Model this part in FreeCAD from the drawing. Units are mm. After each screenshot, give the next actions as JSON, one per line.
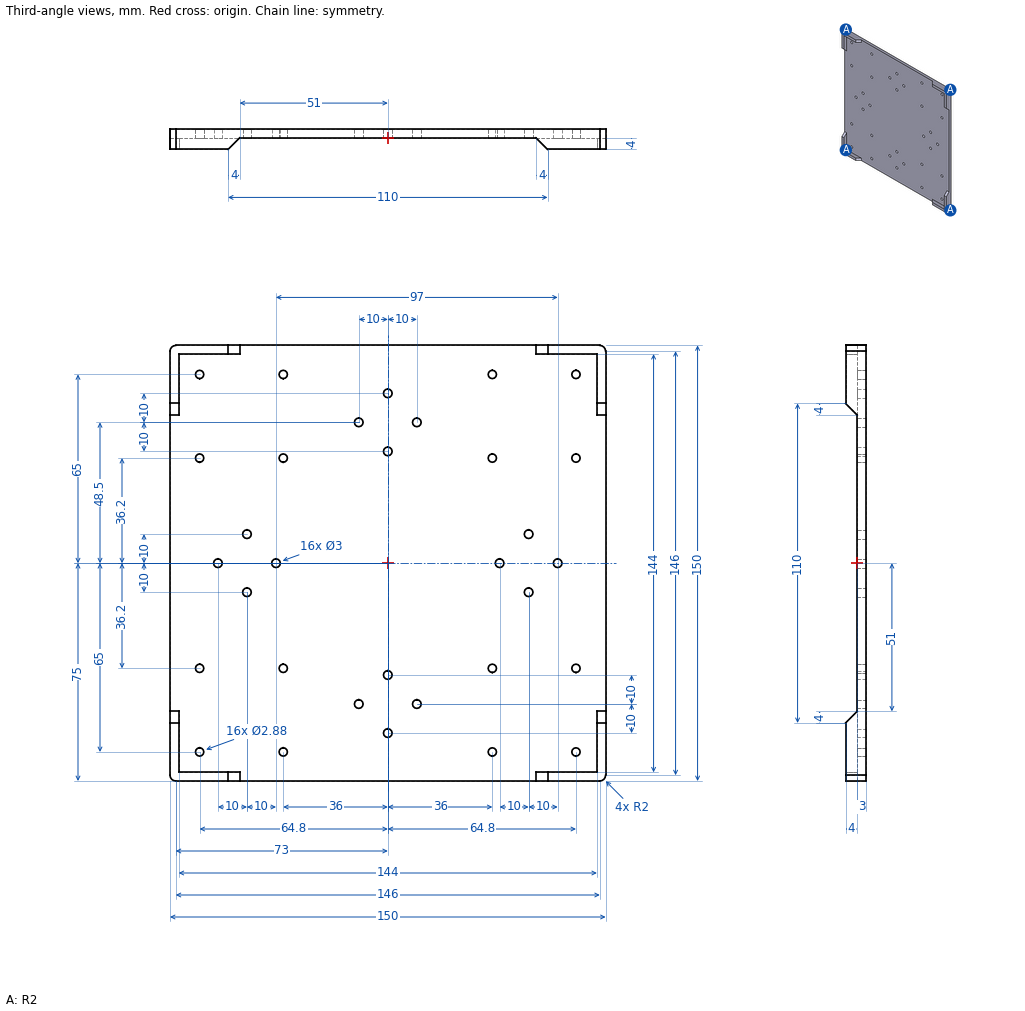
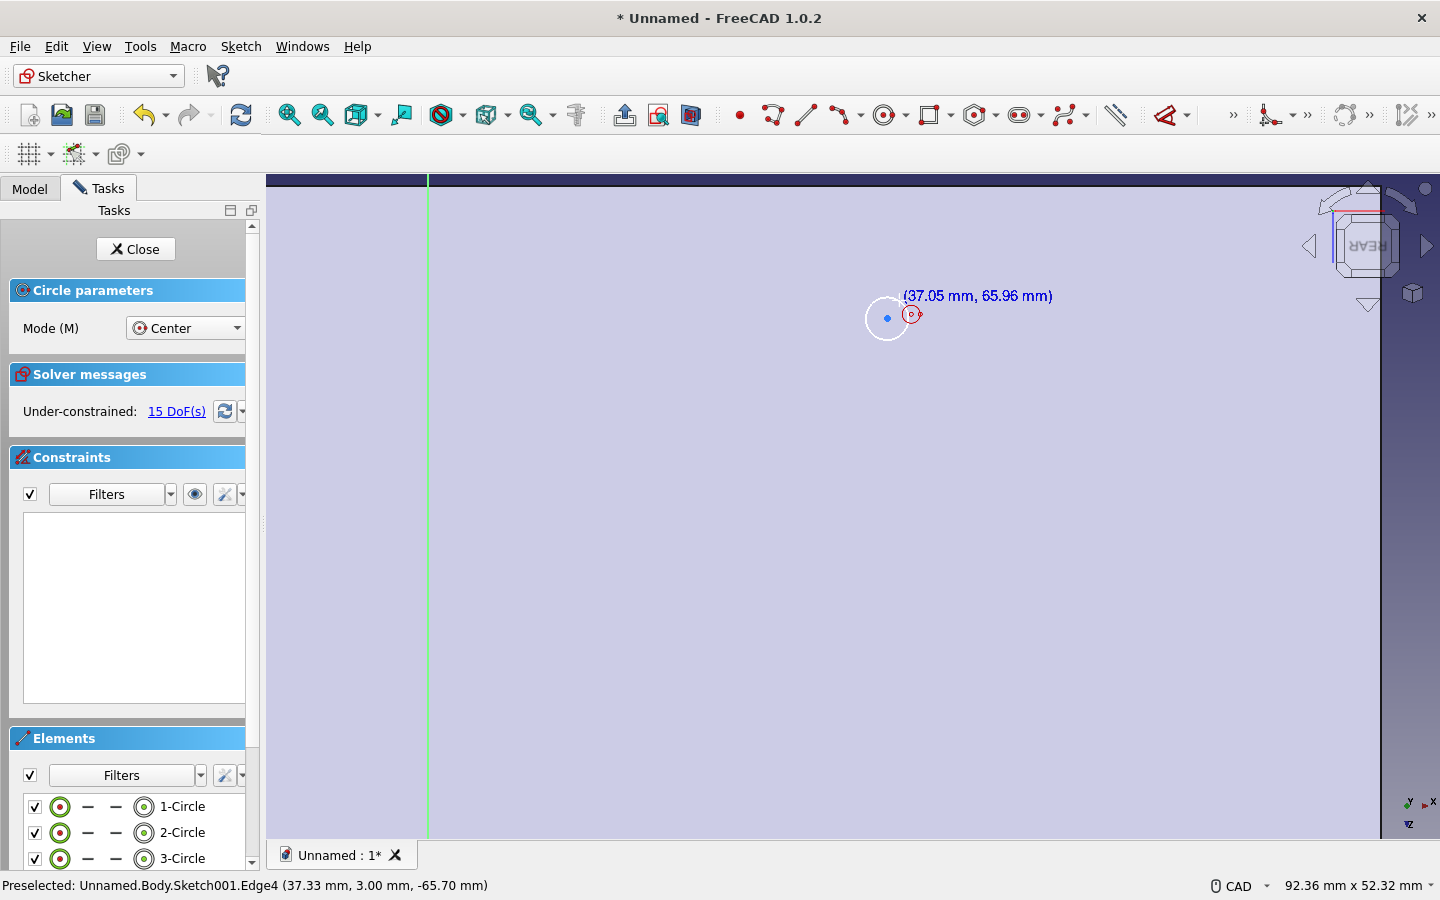
{"action": "scroll", "coordinate": [1252, 313], "scroll_direction": "up", "scroll_amount": 2}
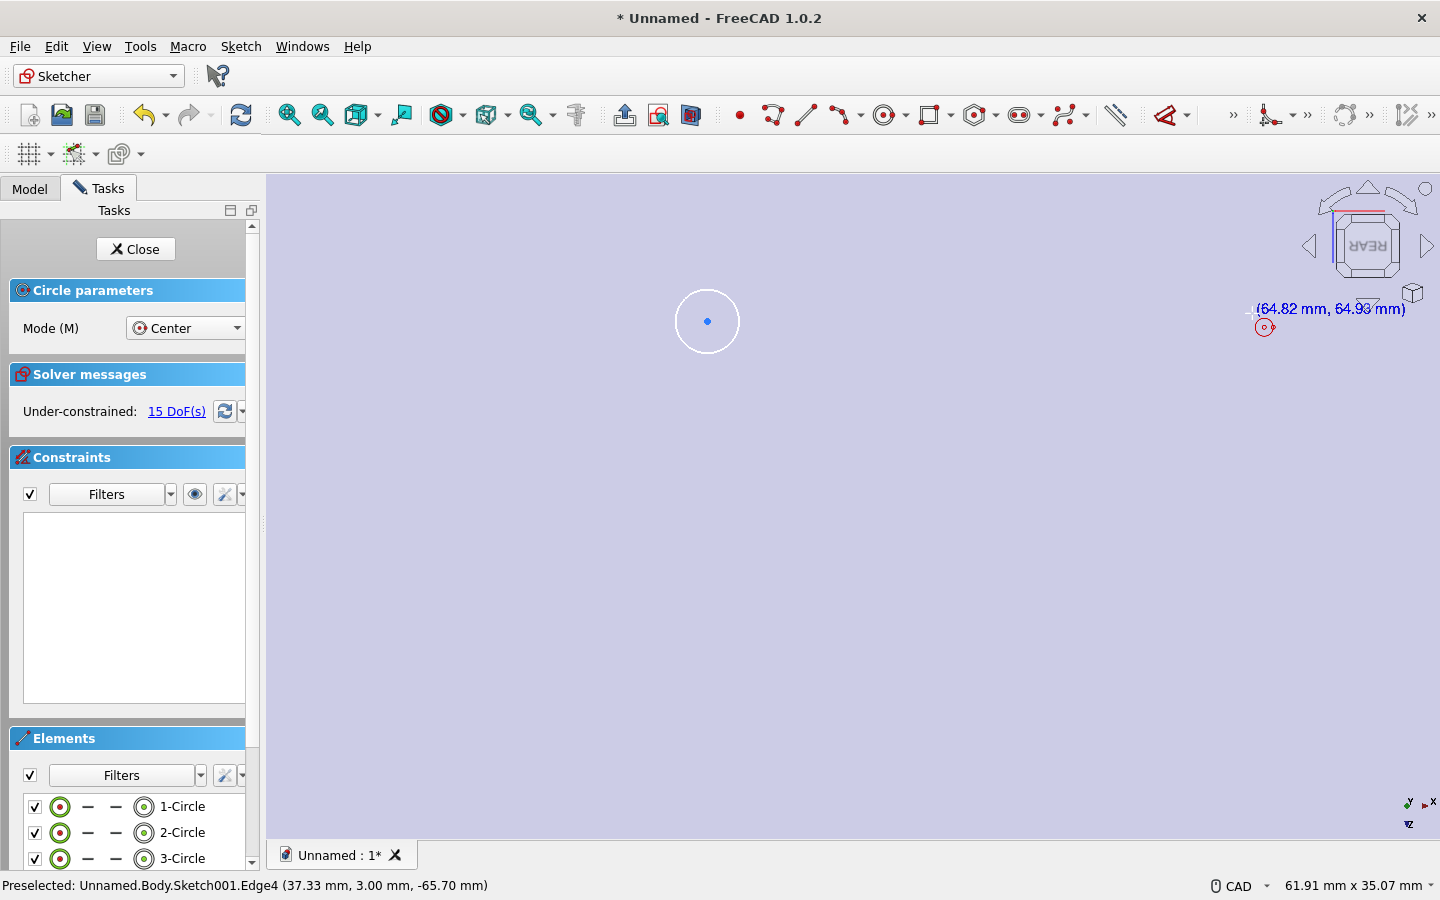
{"action": "scroll", "coordinate": [935, 301], "scroll_direction": "down", "scroll_amount": 9}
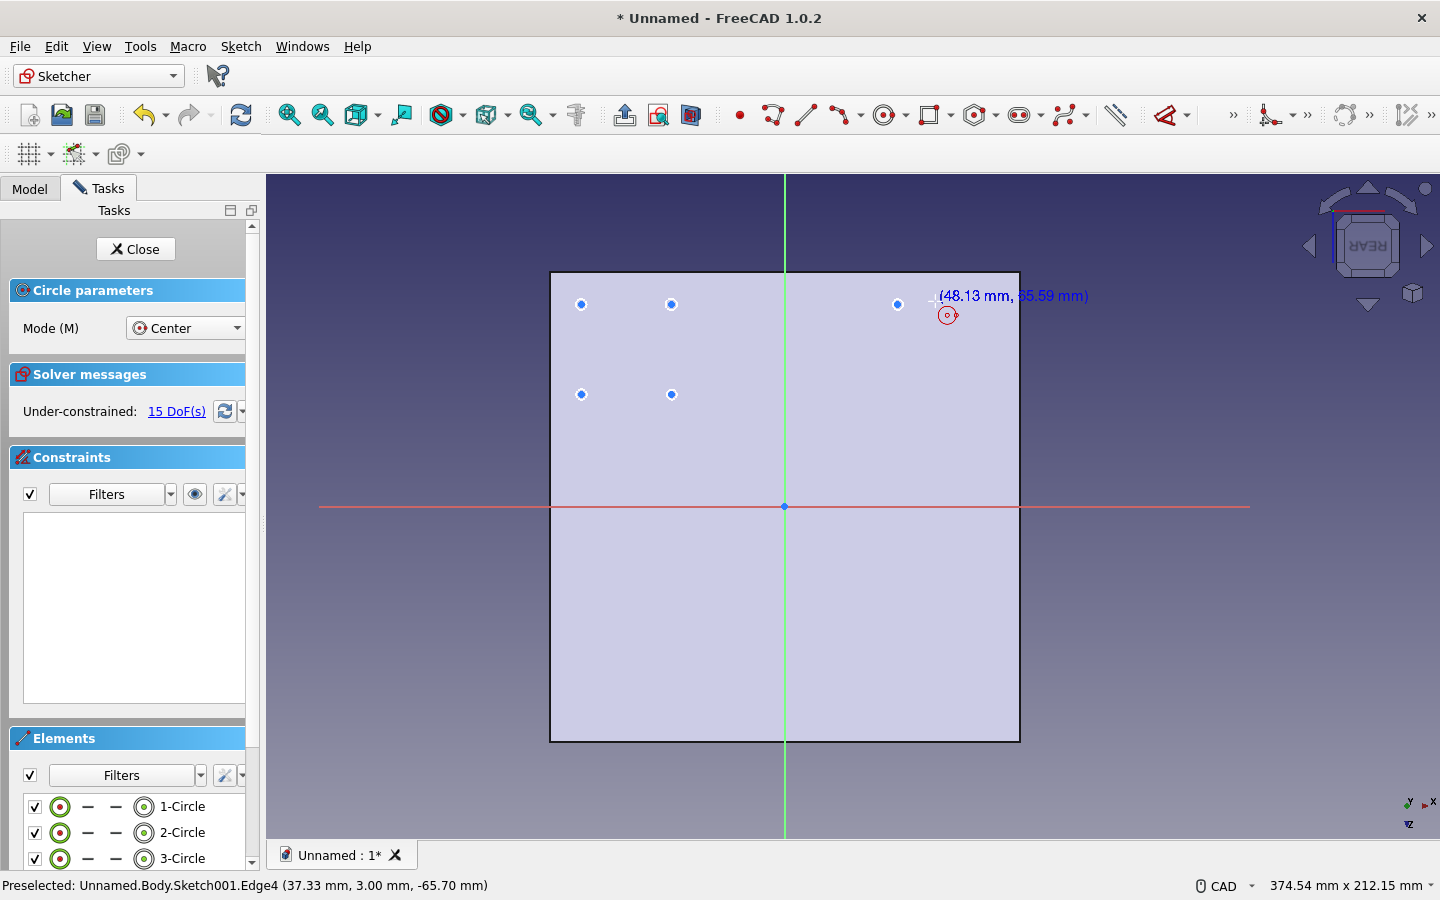
{"action": "left_click", "coordinate": [988, 303]}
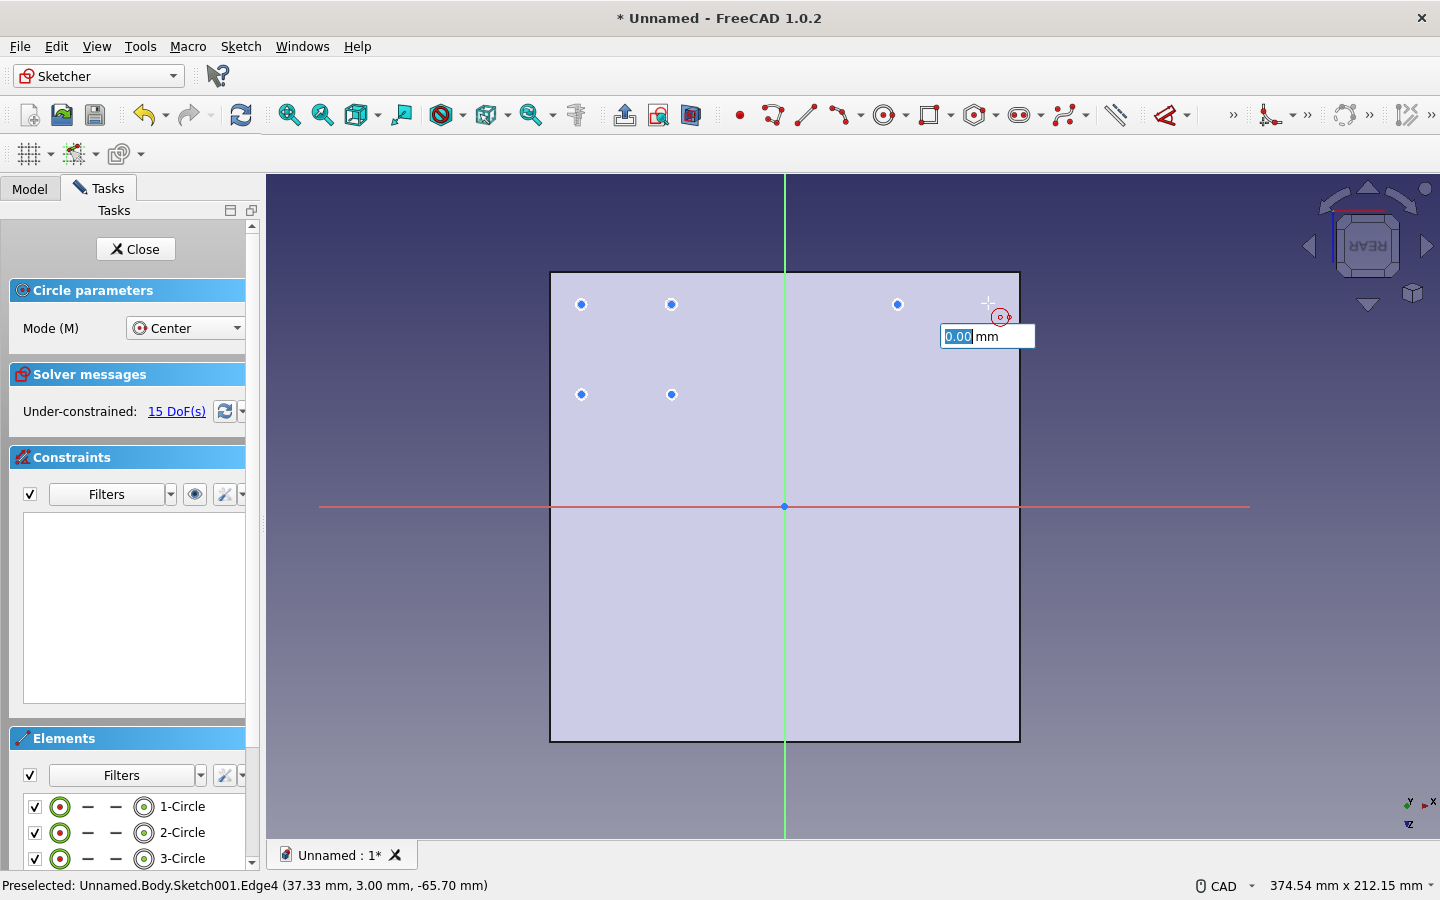
{"action": "scroll", "coordinate": [991, 300], "scroll_direction": "up", "scroll_amount": 7}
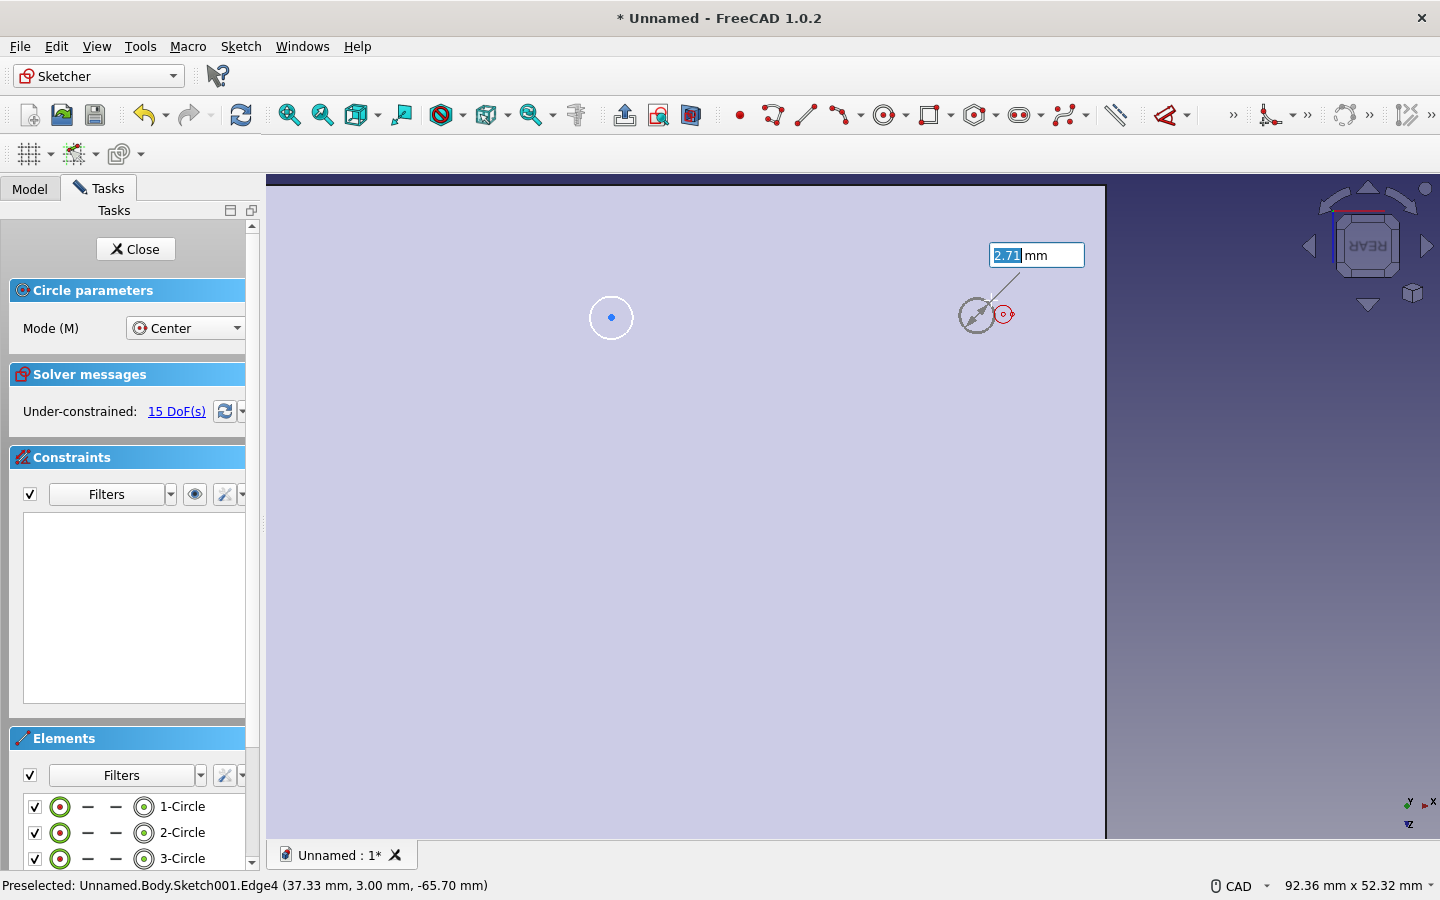
{"action": "left_click", "coordinate": [989, 299]}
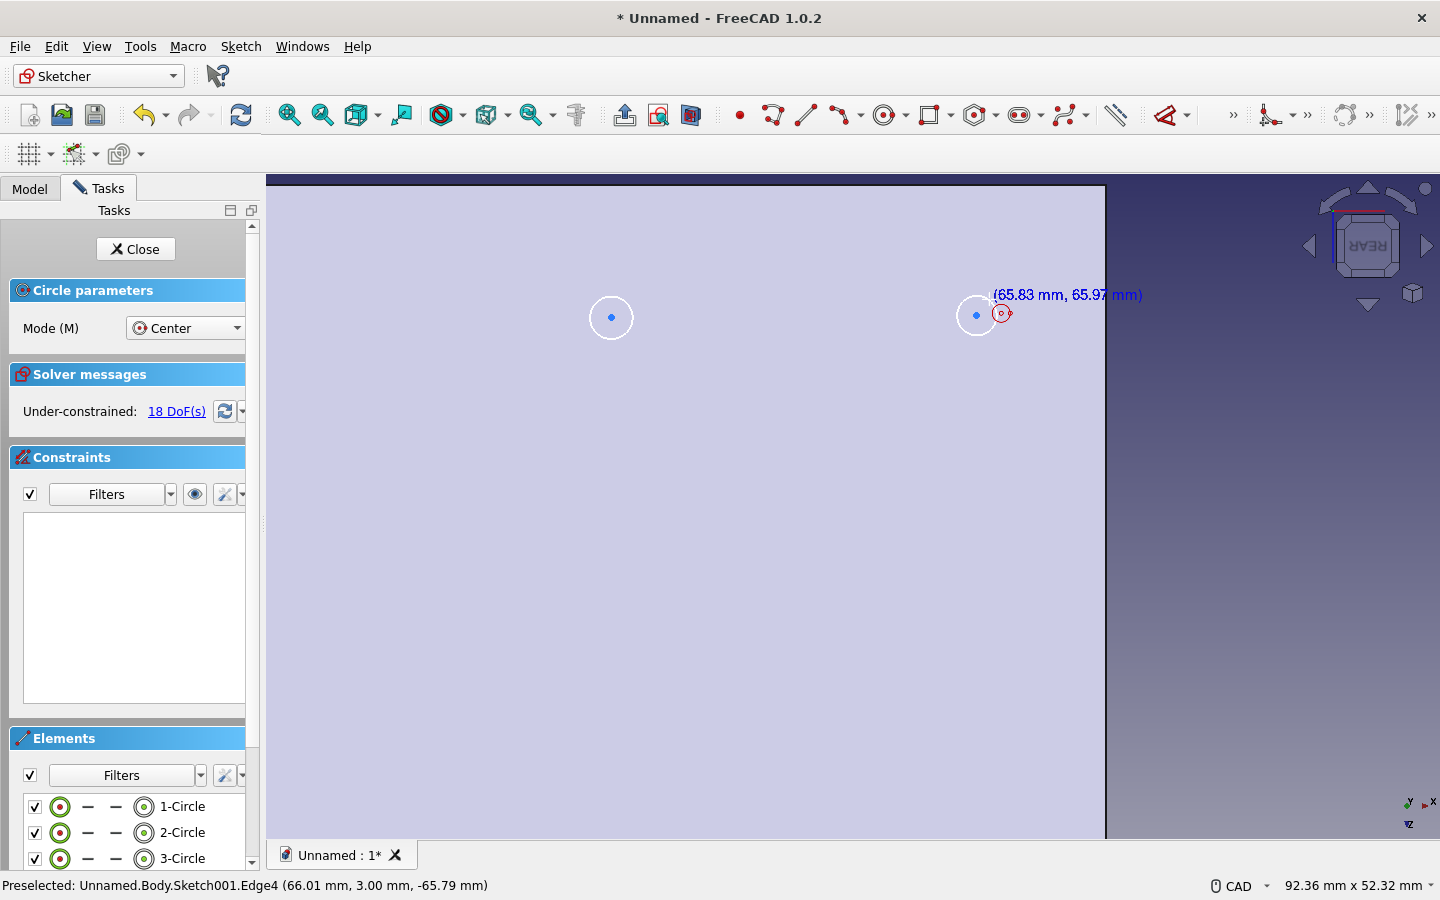
{"action": "scroll", "coordinate": [976, 678], "scroll_direction": "up", "scroll_amount": 2}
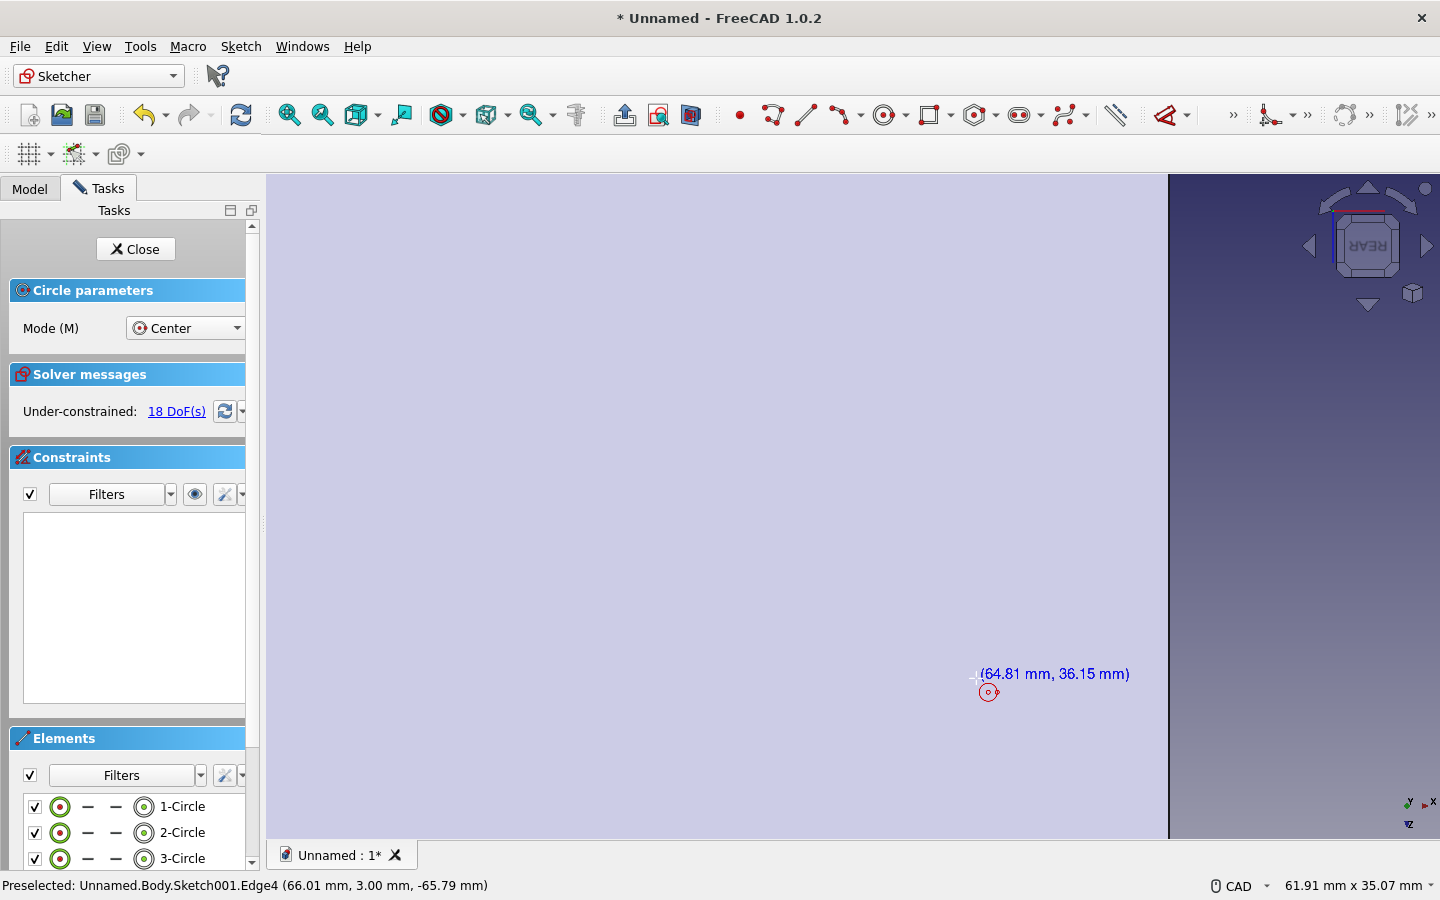
{"action": "scroll", "coordinate": [990, 337], "scroll_direction": "down", "scroll_amount": 9}